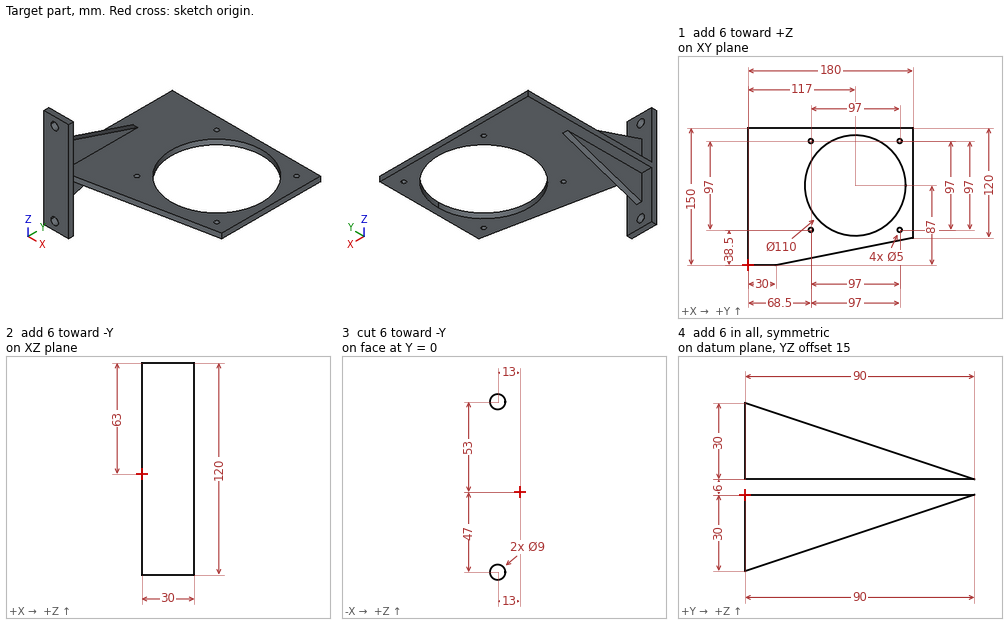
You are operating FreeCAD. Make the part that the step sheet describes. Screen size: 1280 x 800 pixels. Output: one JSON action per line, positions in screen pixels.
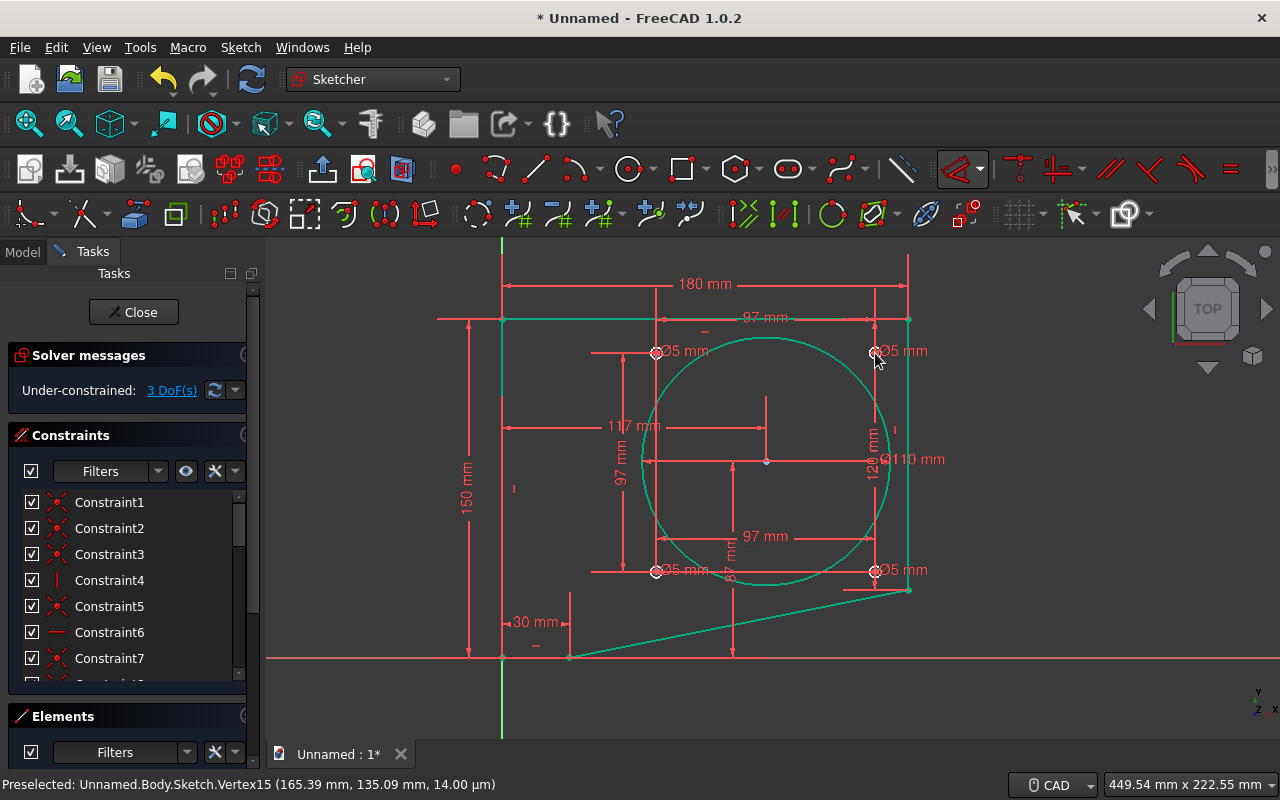
{"action": "left_click", "coordinate": [982, 170]}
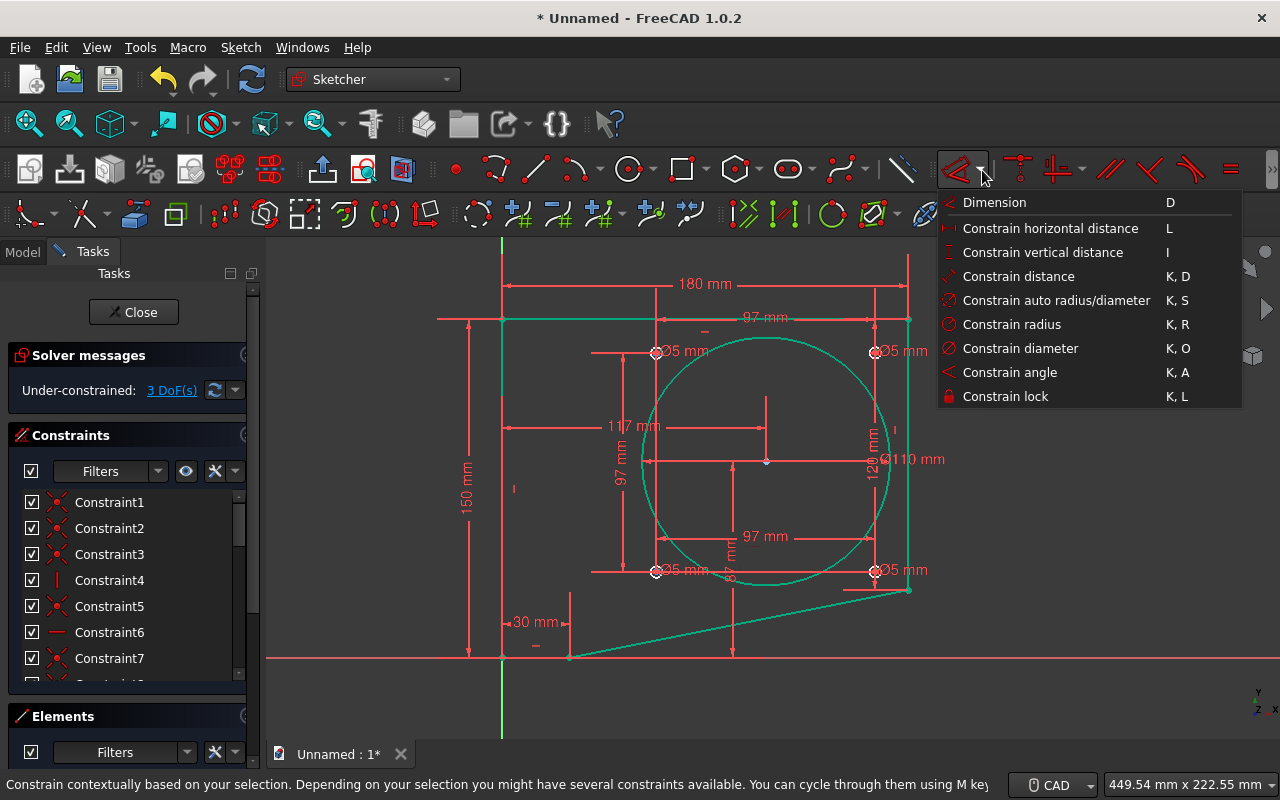
{"action": "left_click", "coordinate": [1090, 252]}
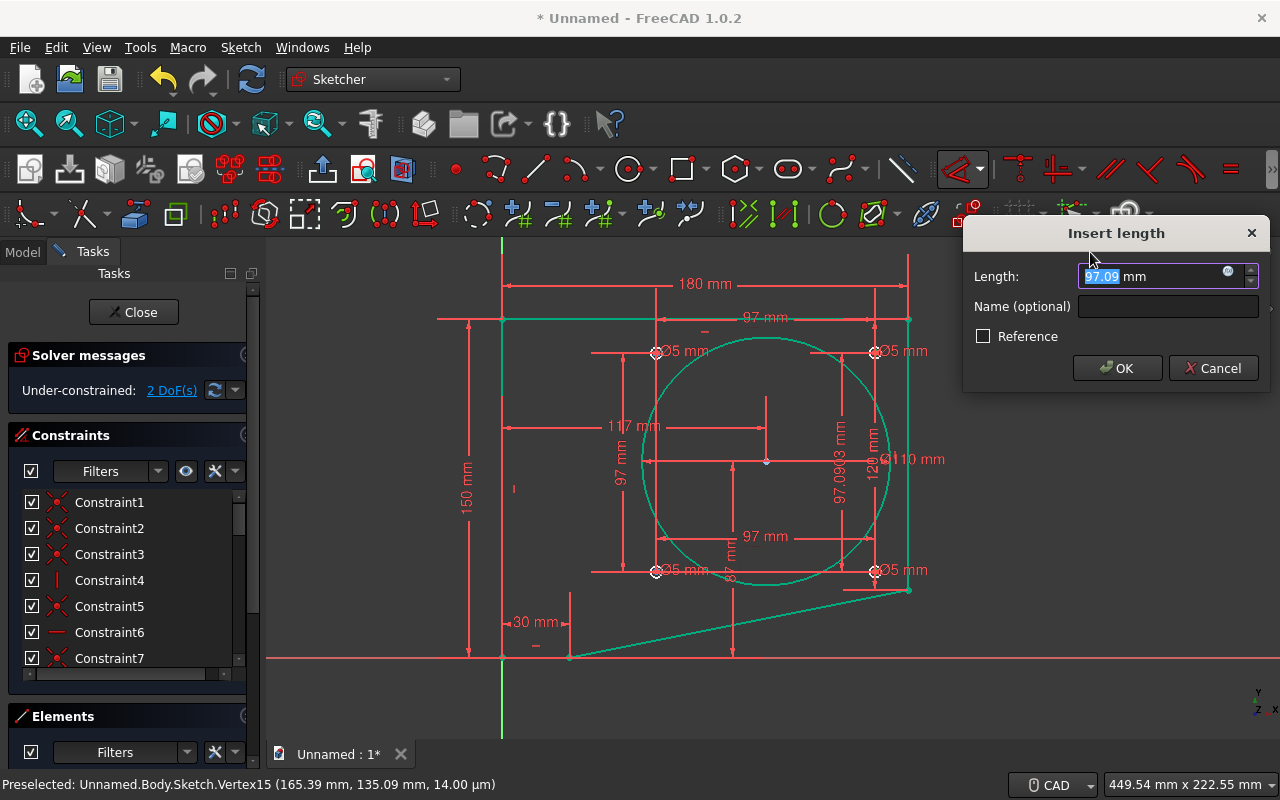
{"action": "type", "text": "97"}
{"action": "key", "text": "Return"}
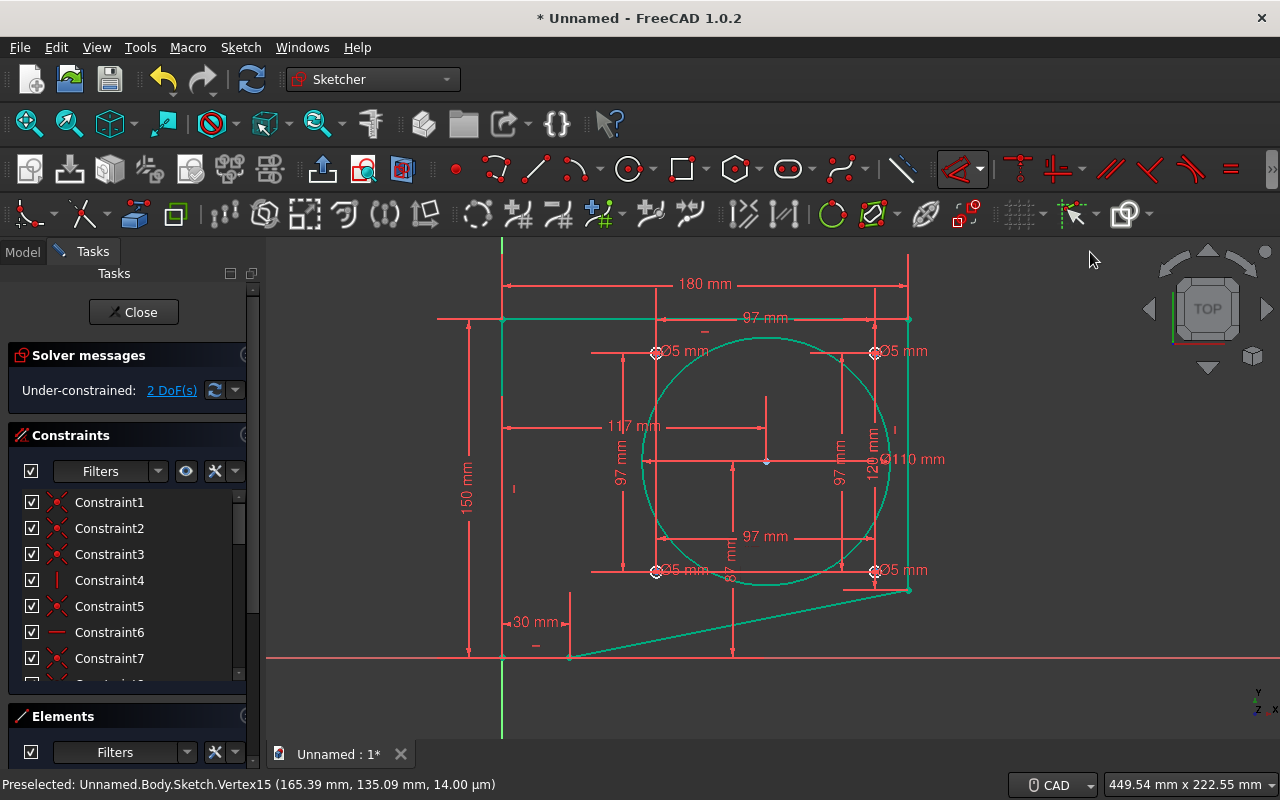
{"action": "left_click", "coordinate": [656, 572]}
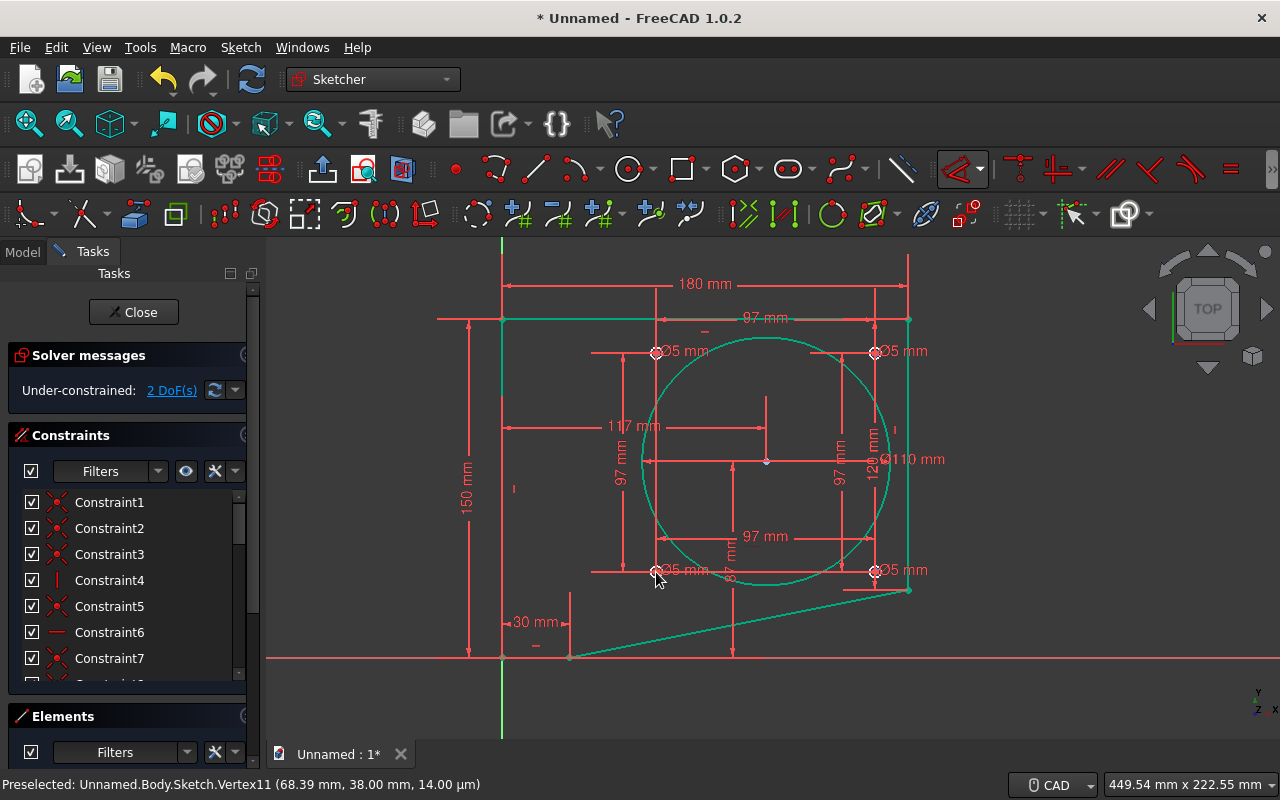
{"action": "left_click", "coordinate": [982, 170]}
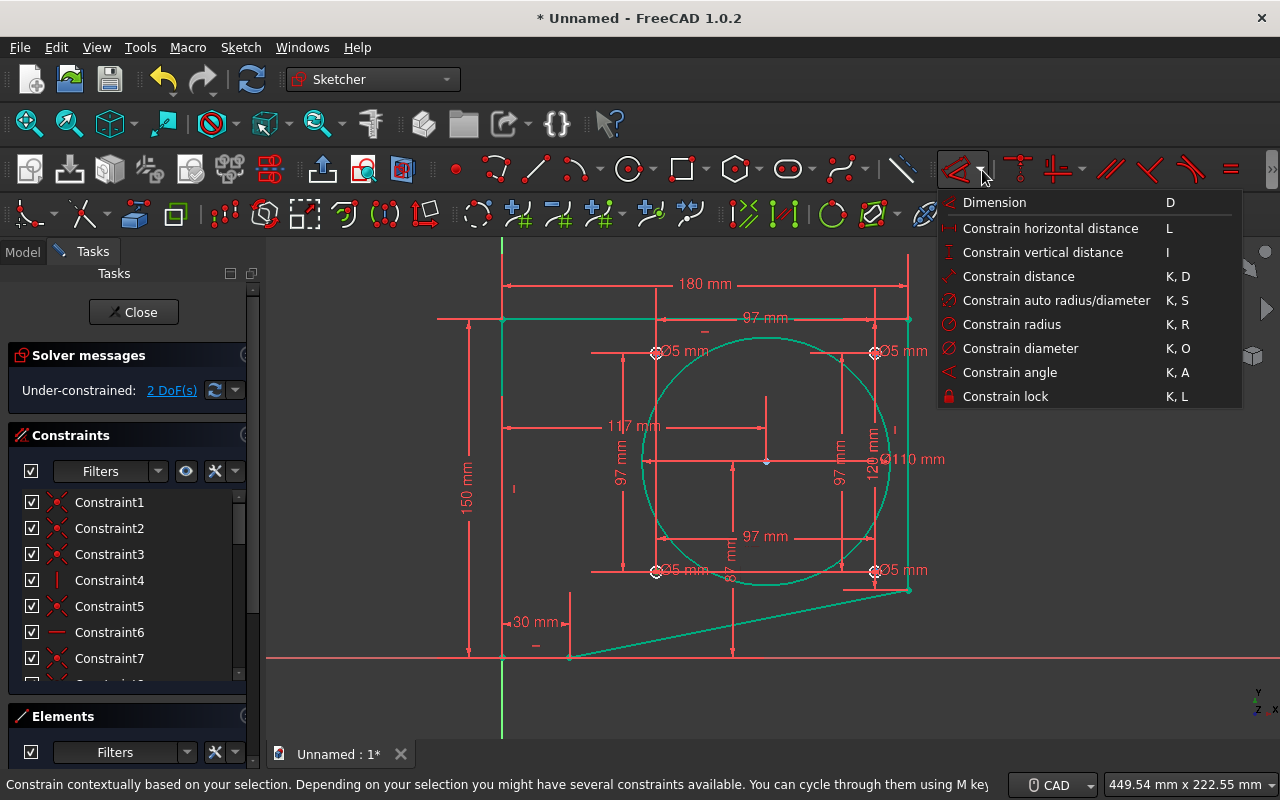
{"action": "left_click", "coordinate": [1090, 228]}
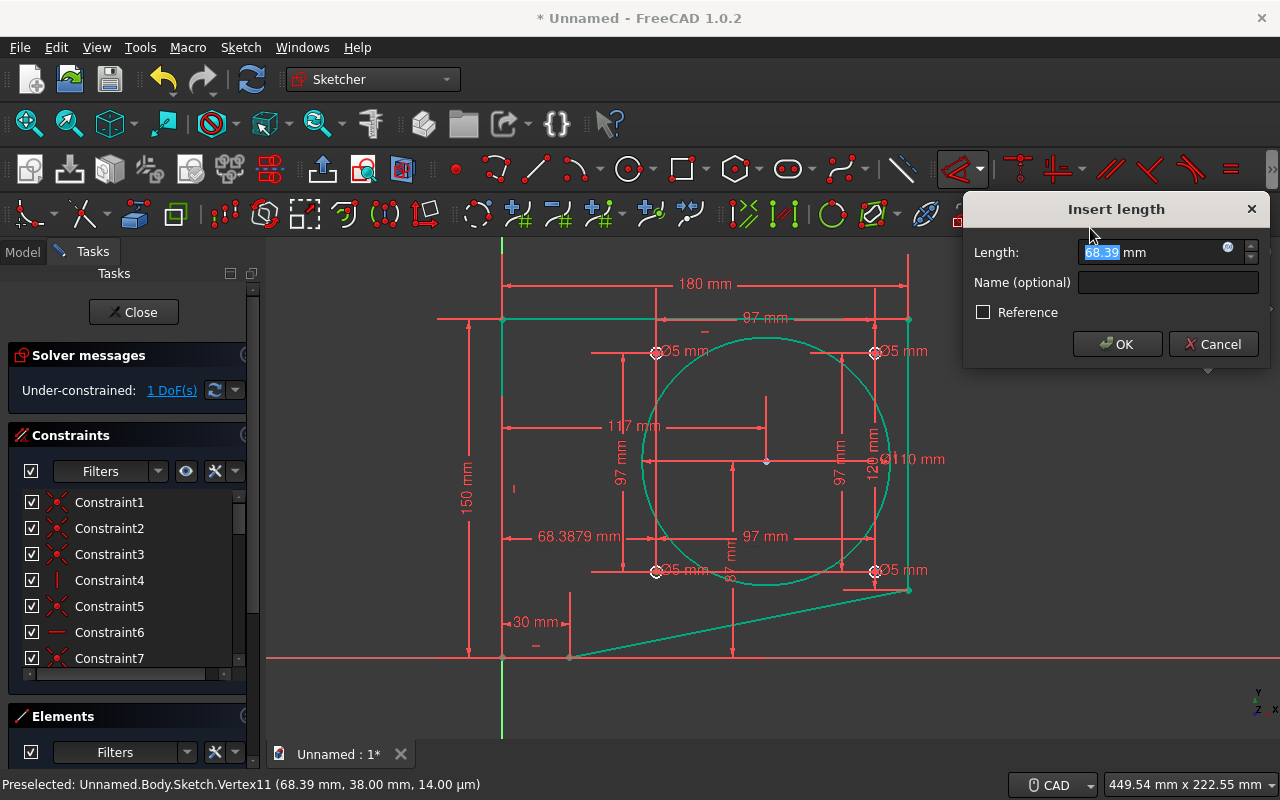
{"action": "type", "text": "68.5"}
{"action": "key", "text": "Return"}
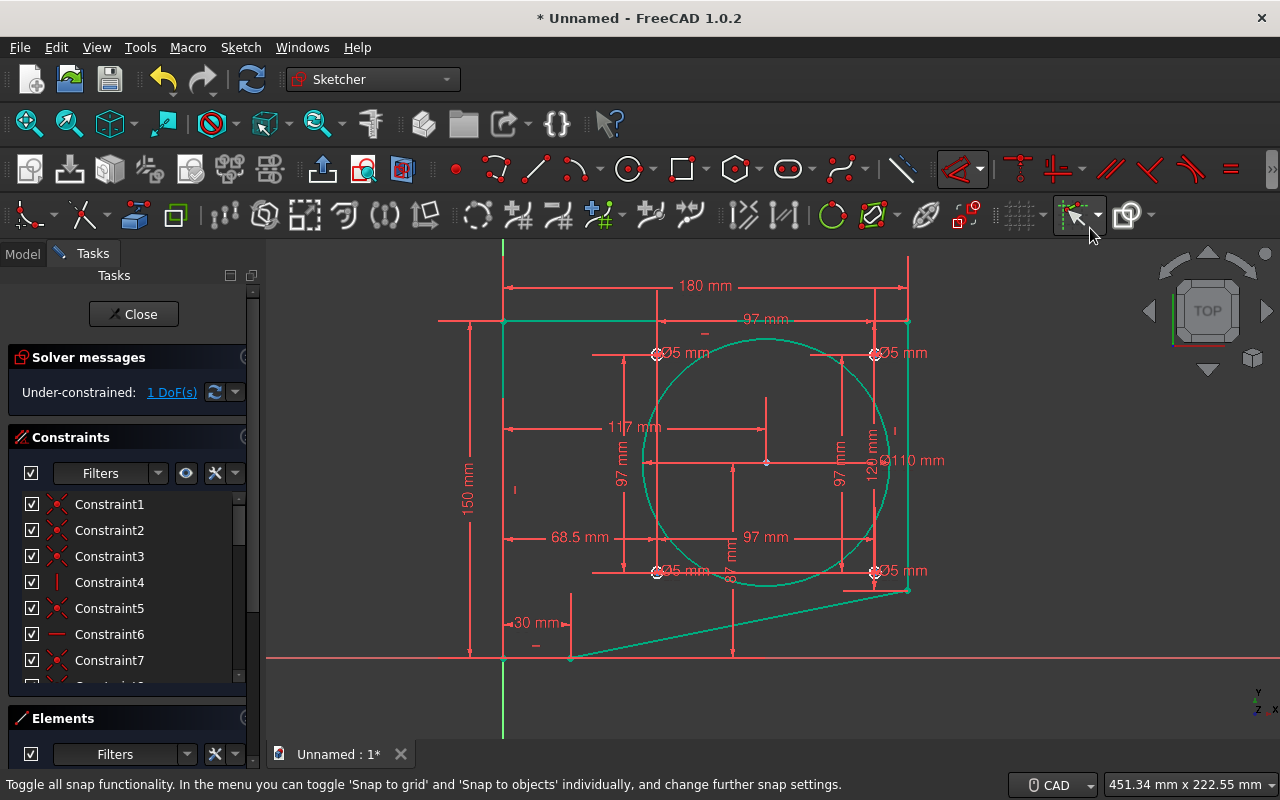
{"action": "left_click", "coordinate": [657, 573]}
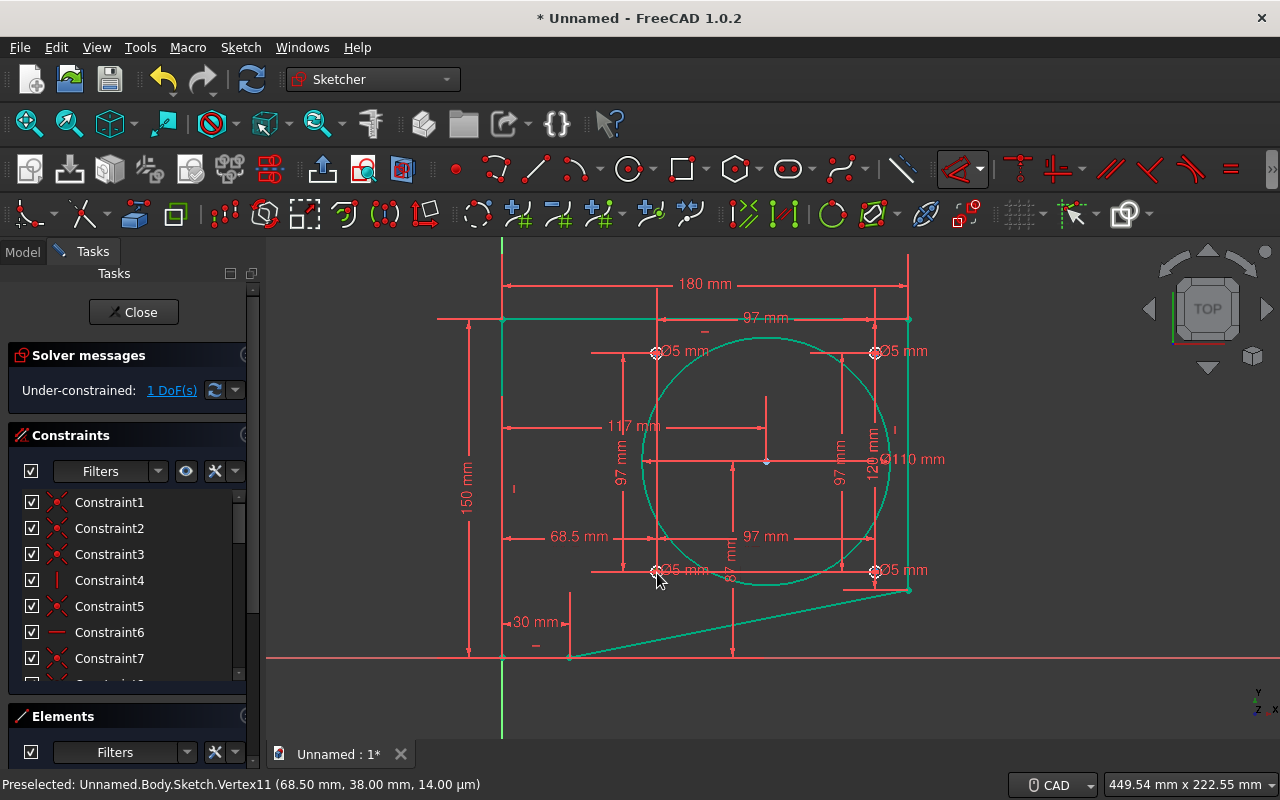
{"action": "key", "text": "i"}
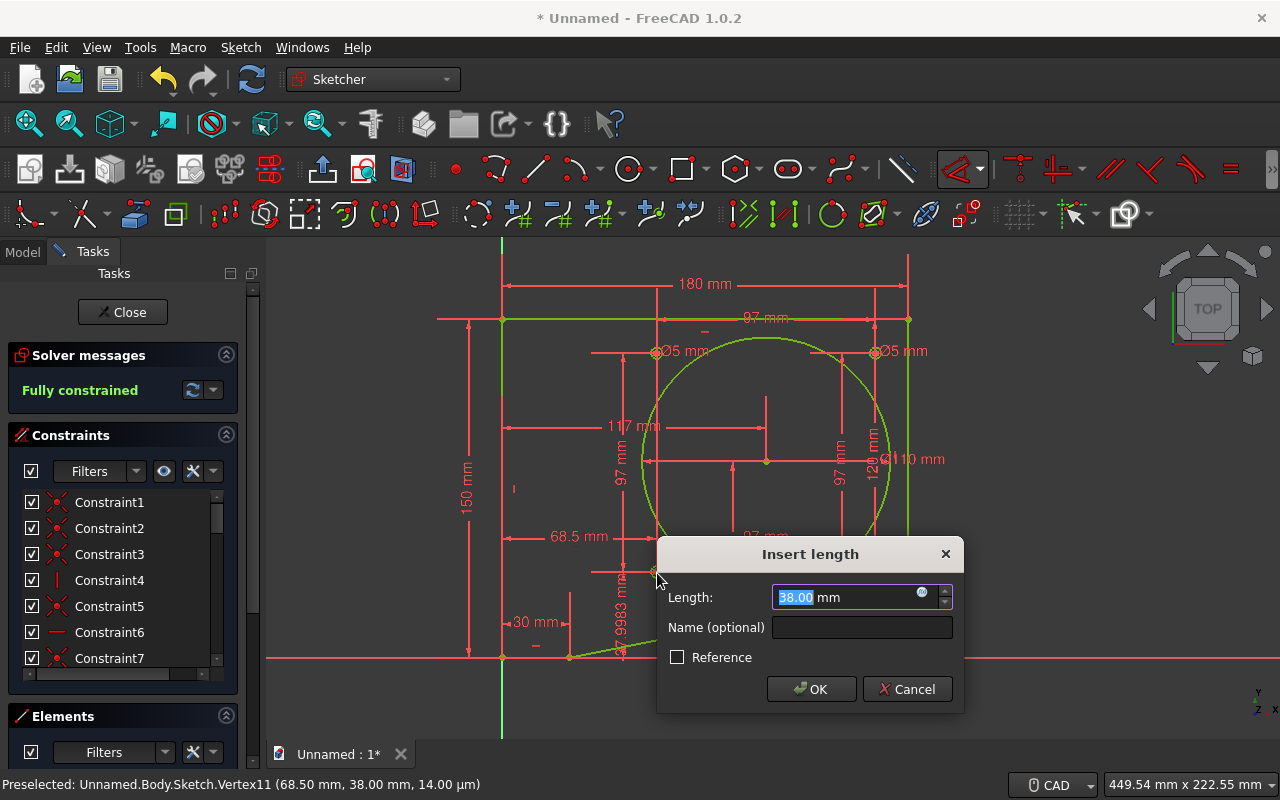
{"action": "type", "text": "38.5"}
{"action": "key", "text": "Return"}